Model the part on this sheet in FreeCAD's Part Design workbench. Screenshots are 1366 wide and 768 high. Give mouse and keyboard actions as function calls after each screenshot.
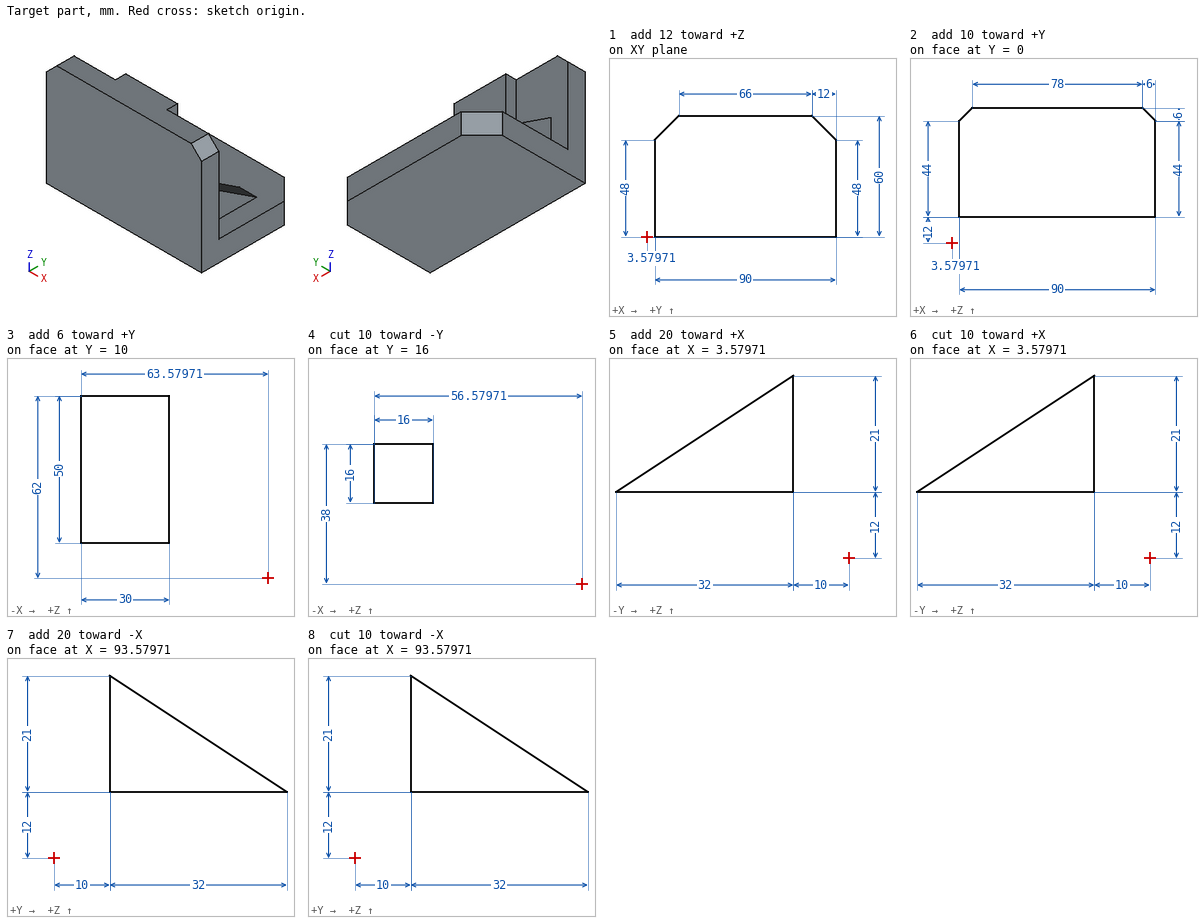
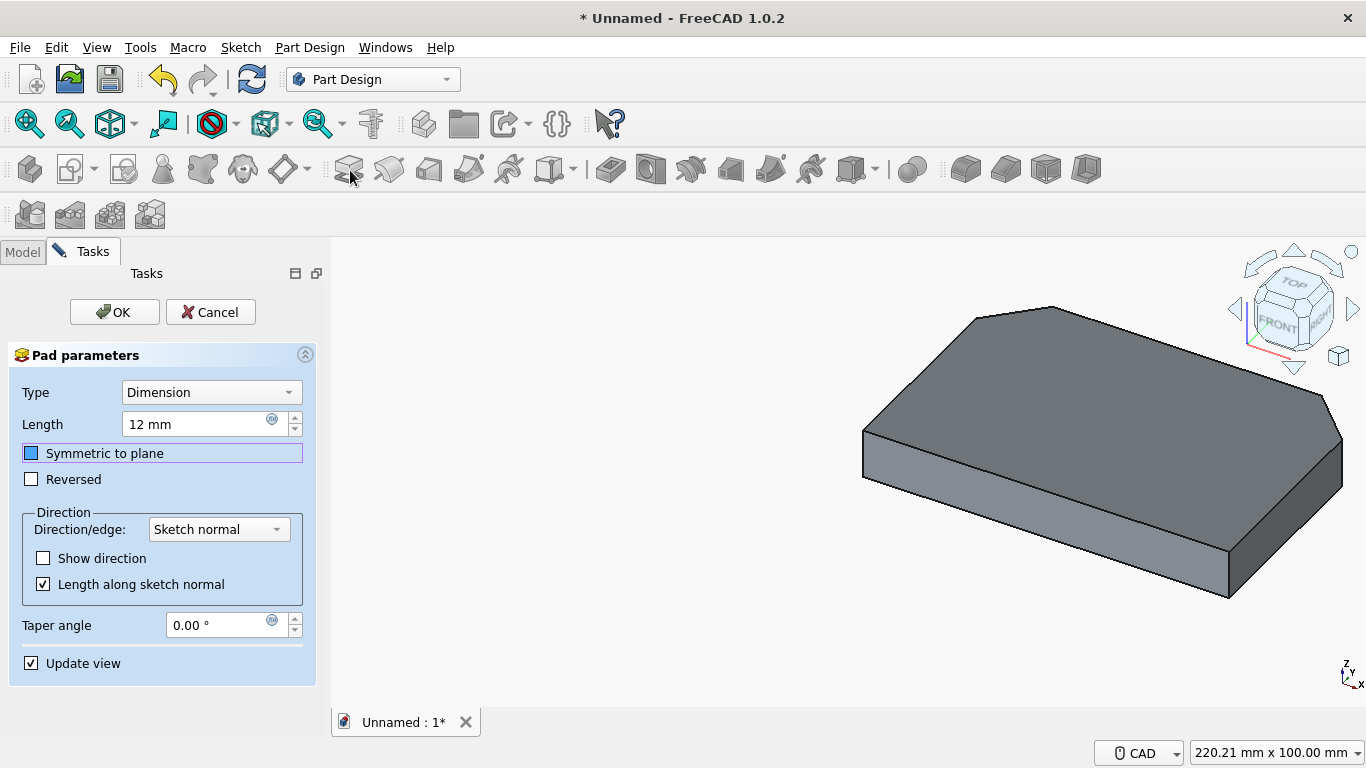
click(115, 312)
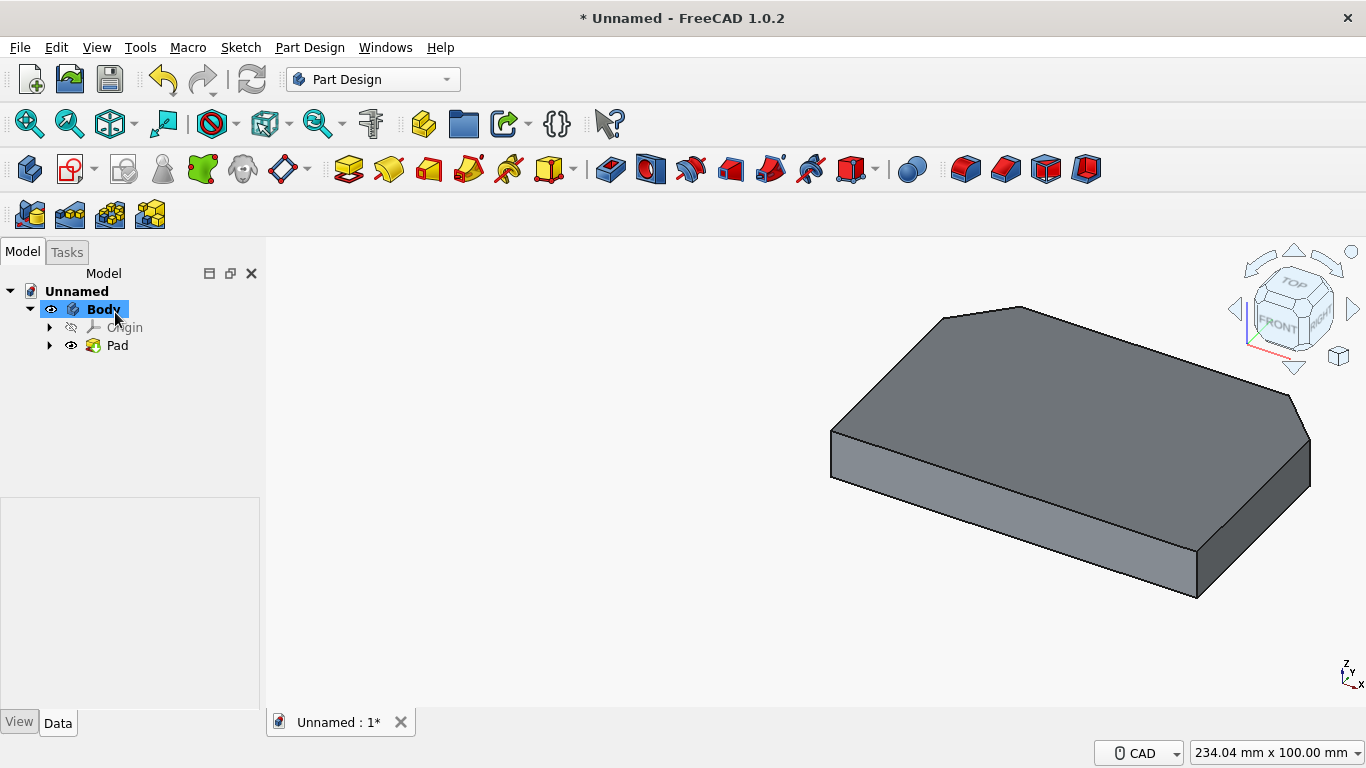
click(1171, 565)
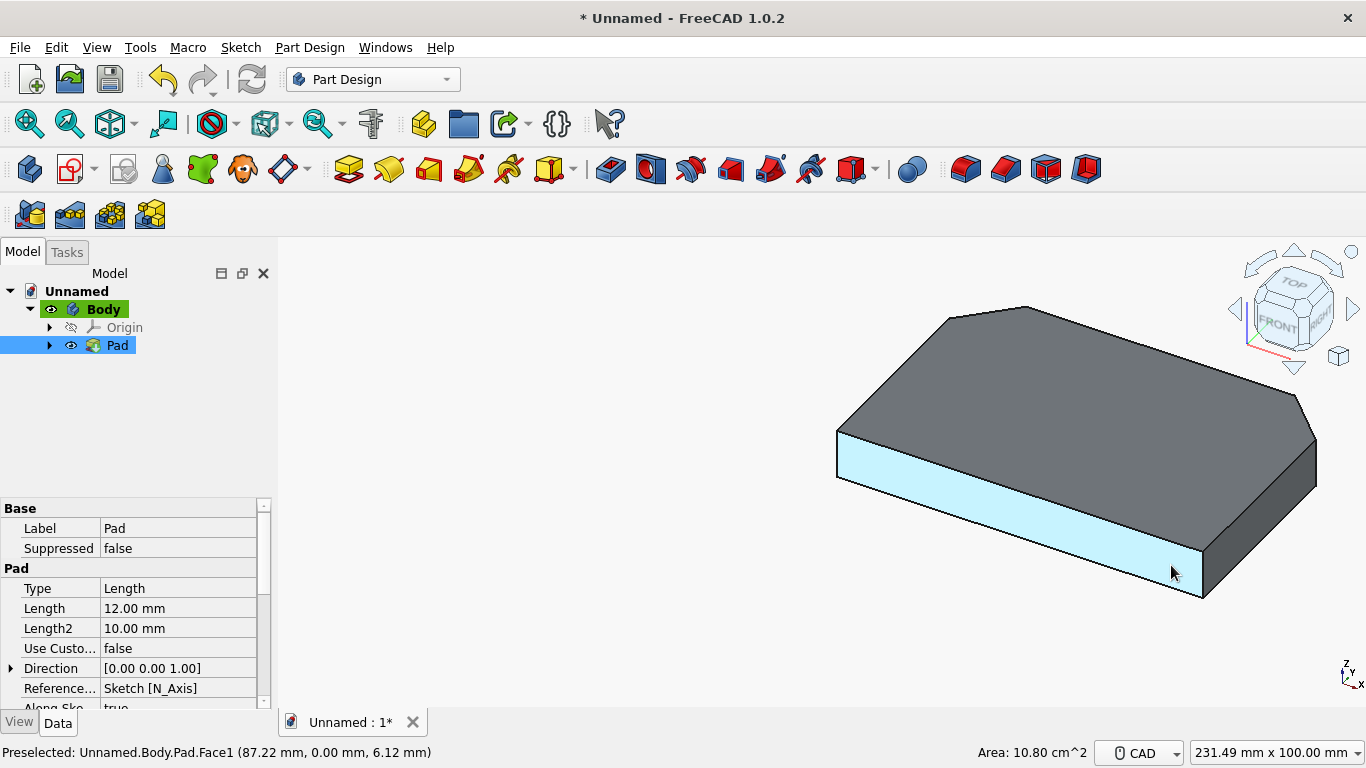
click(70, 170)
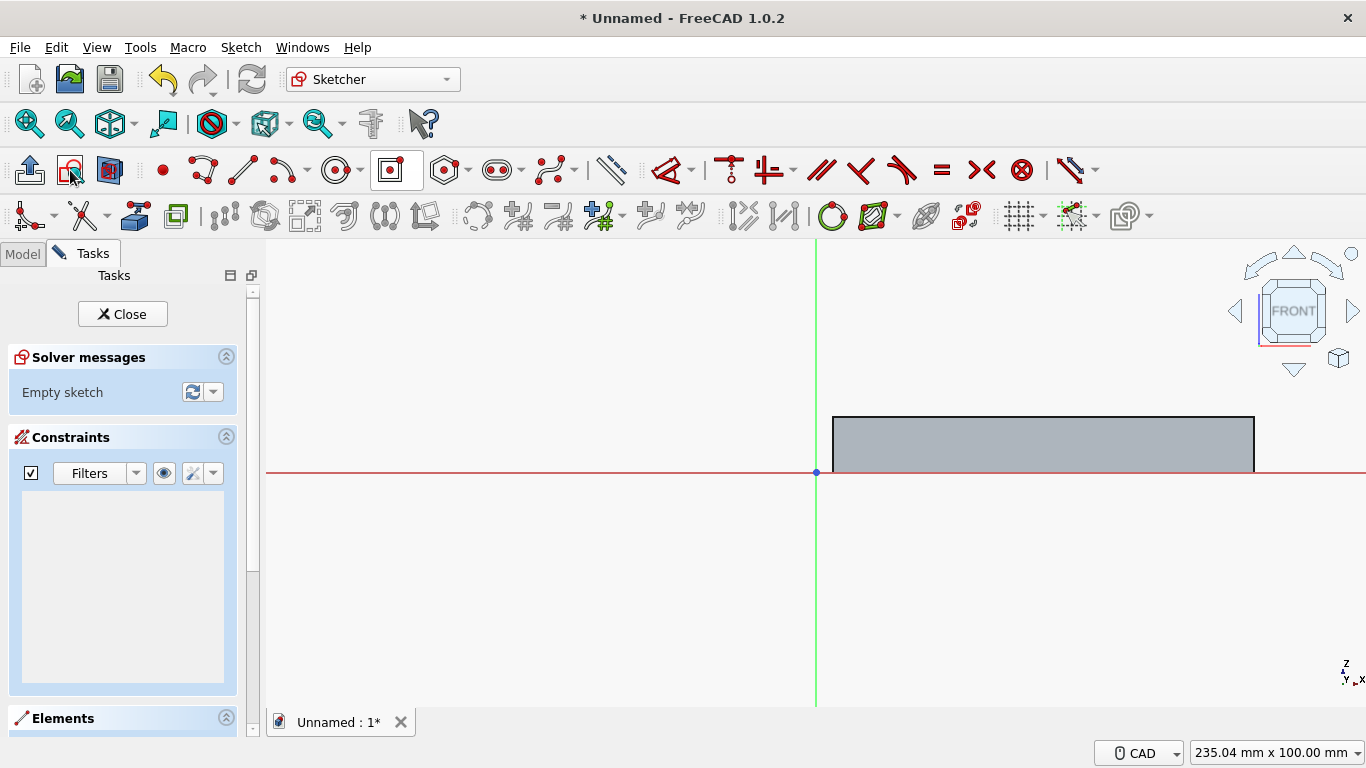
scroll(294, 679, down, 2)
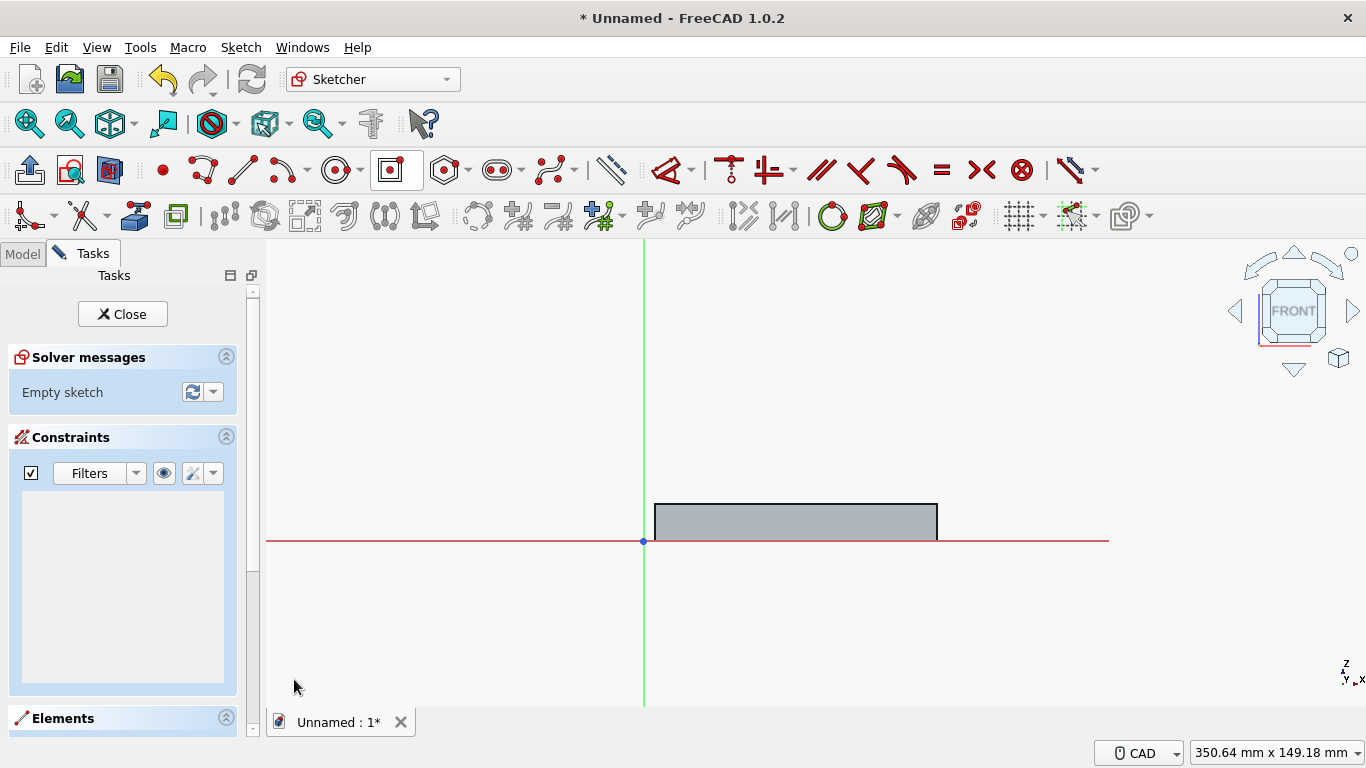
scroll(879, 385, up, 2)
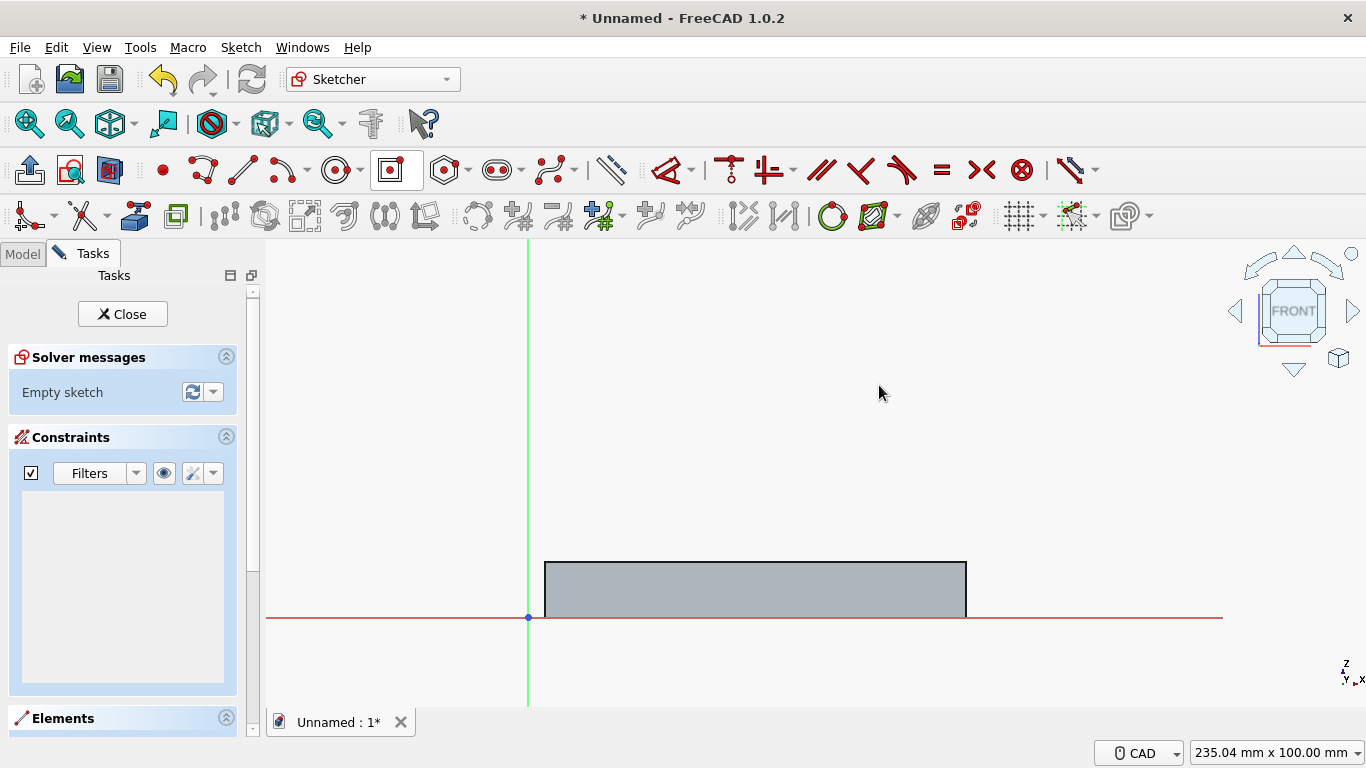
click(204, 170)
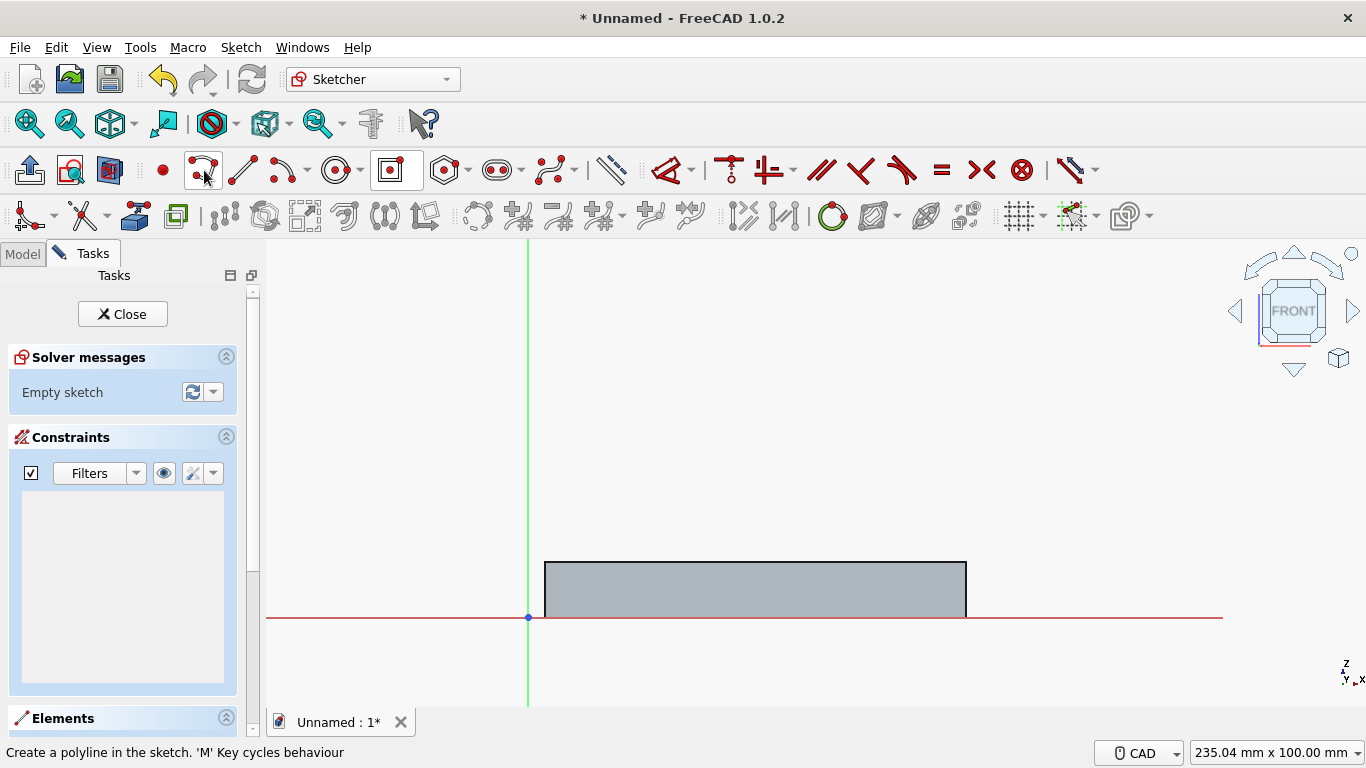
click(545, 562)
click(966, 562)
click(966, 356)
click(938, 328)
click(573, 328)
click(545, 356)
click(545, 563)
key(Escape)
key(Escape)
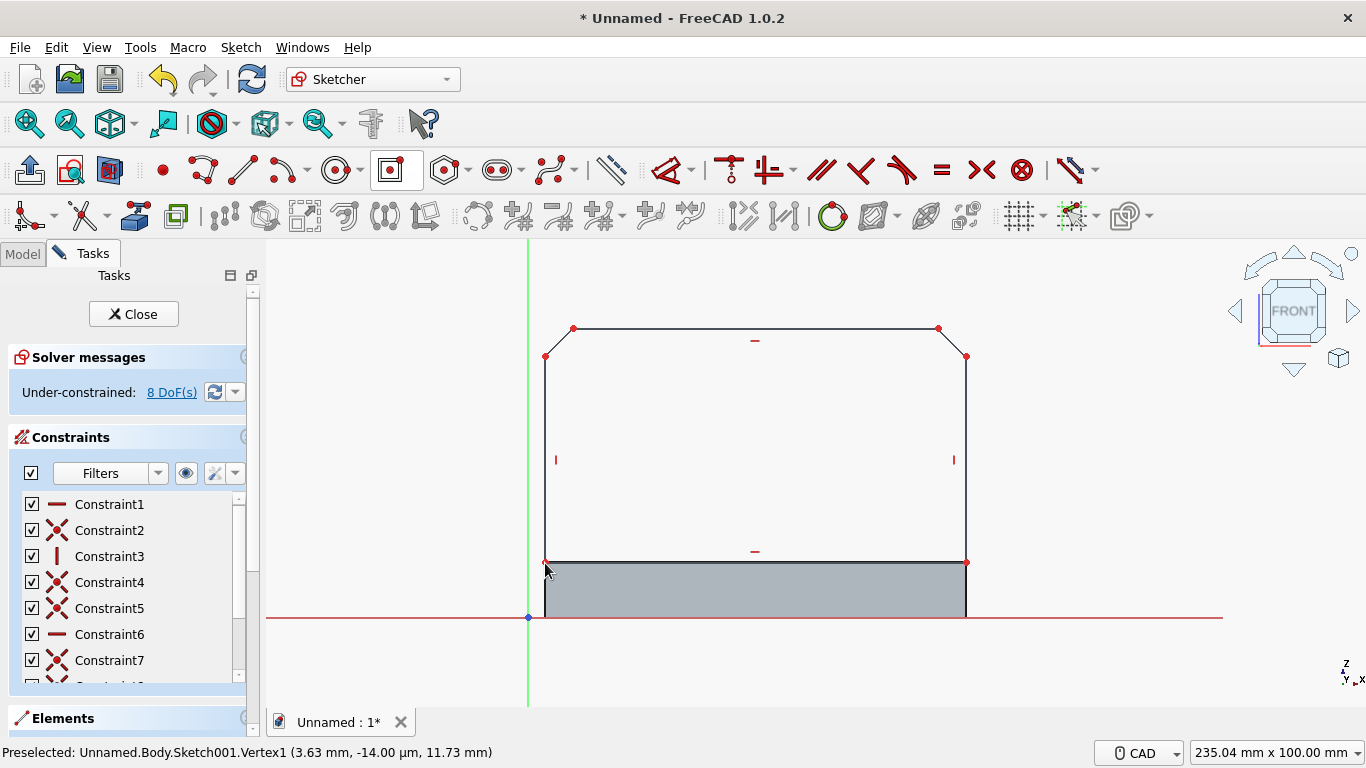
key(d)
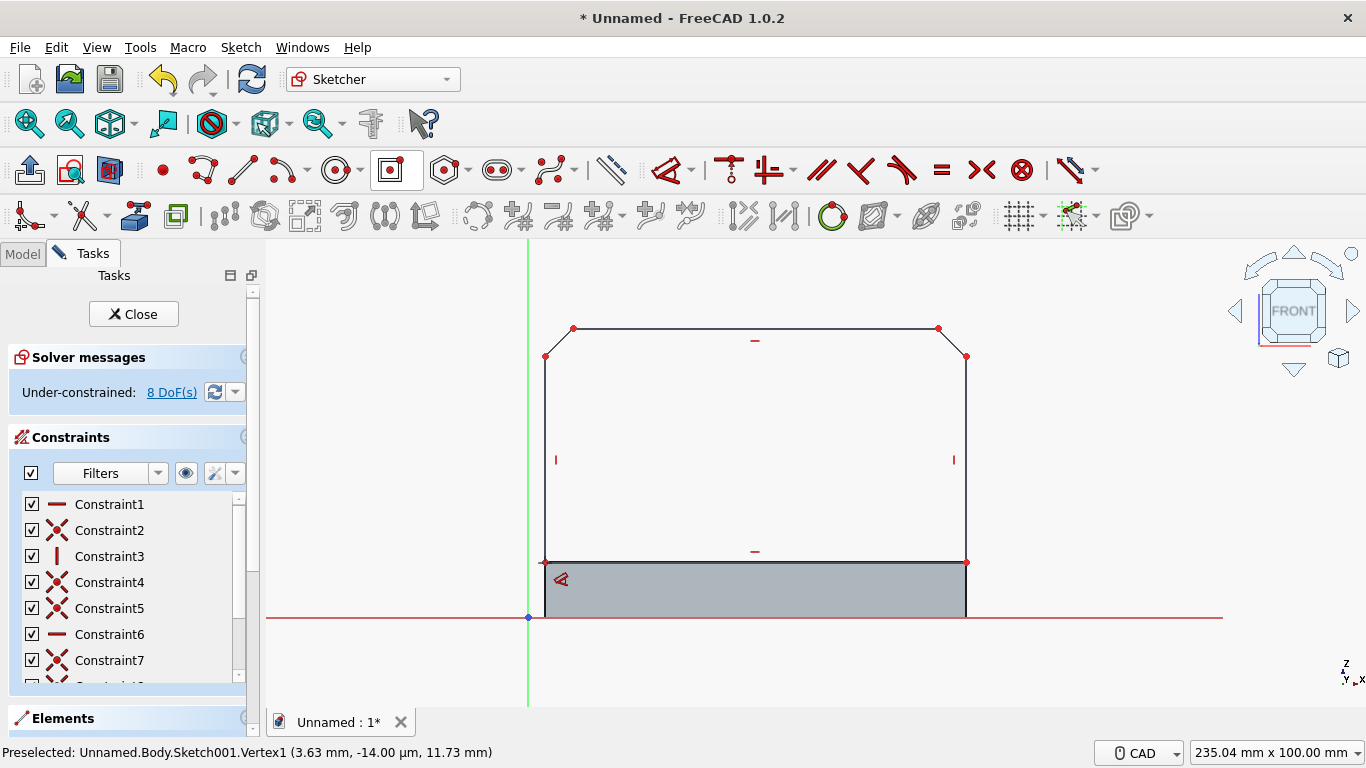
click(671, 563)
click(755, 597)